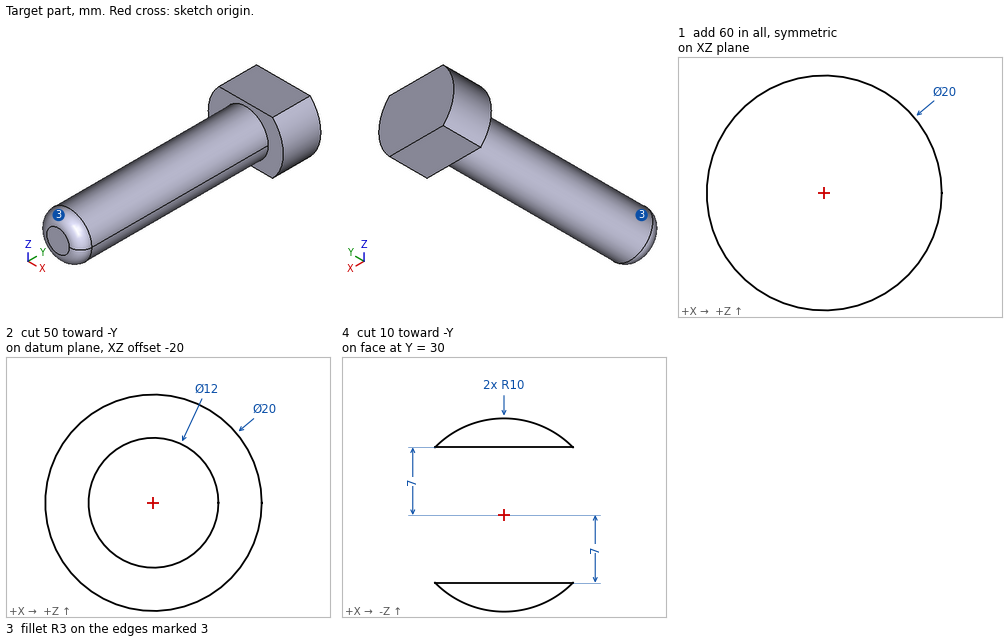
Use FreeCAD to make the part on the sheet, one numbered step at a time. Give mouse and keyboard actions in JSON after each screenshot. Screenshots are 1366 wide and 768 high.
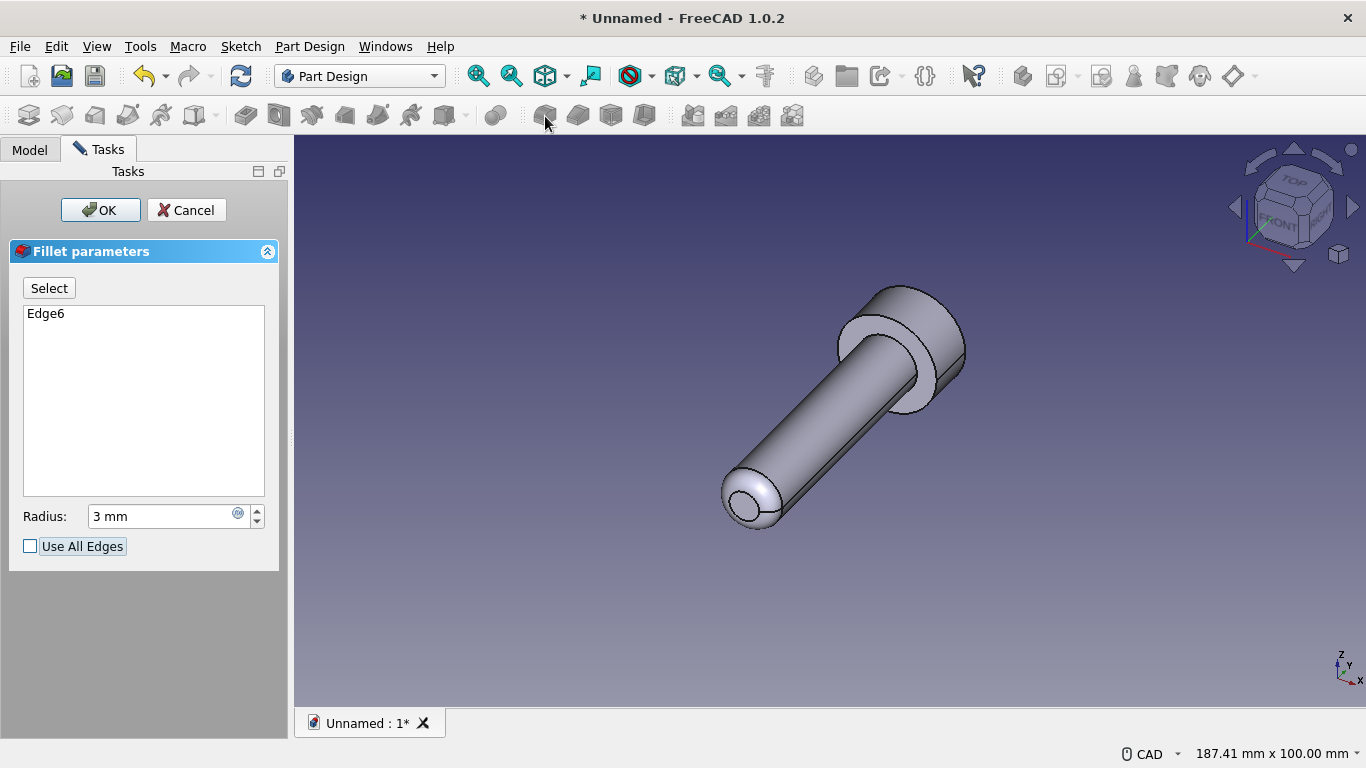
{"action": "left_click", "coordinate": [101, 210]}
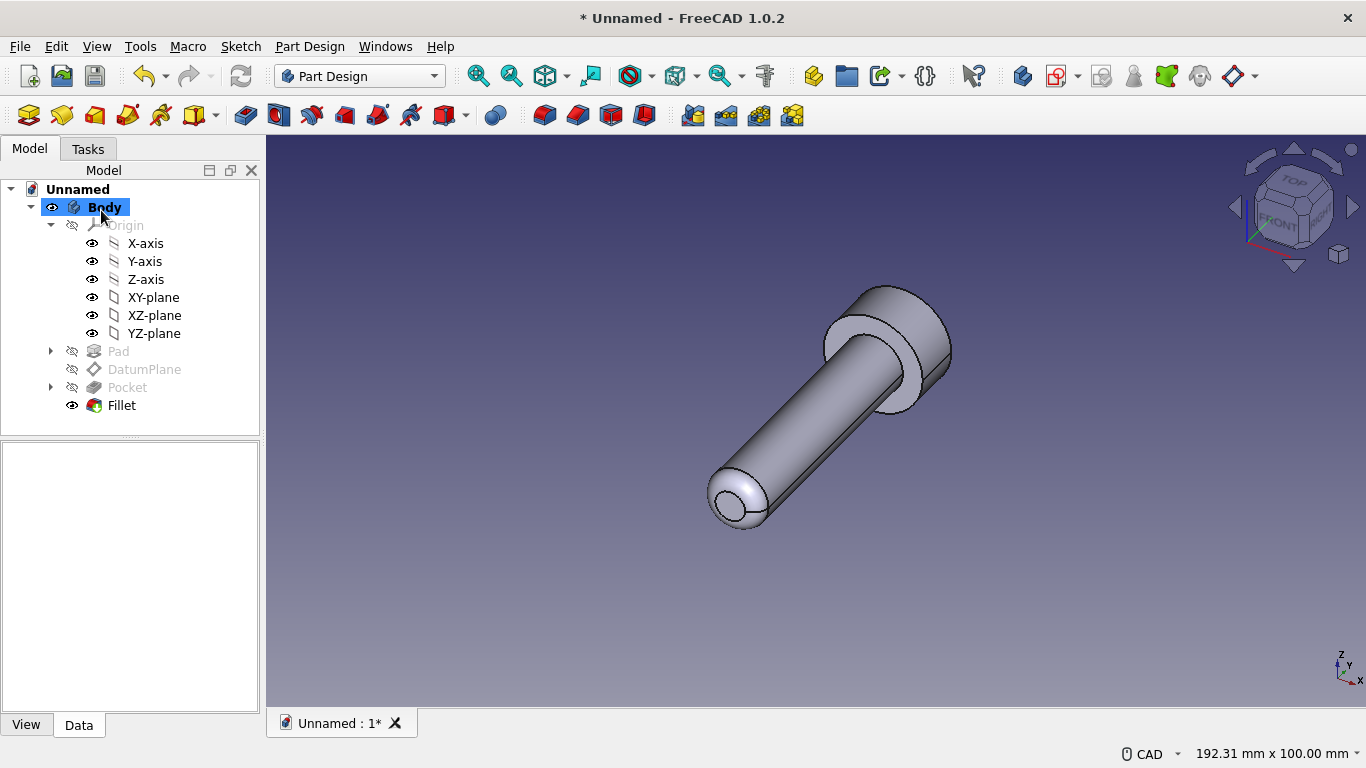
{"action": "key", "text": "4"}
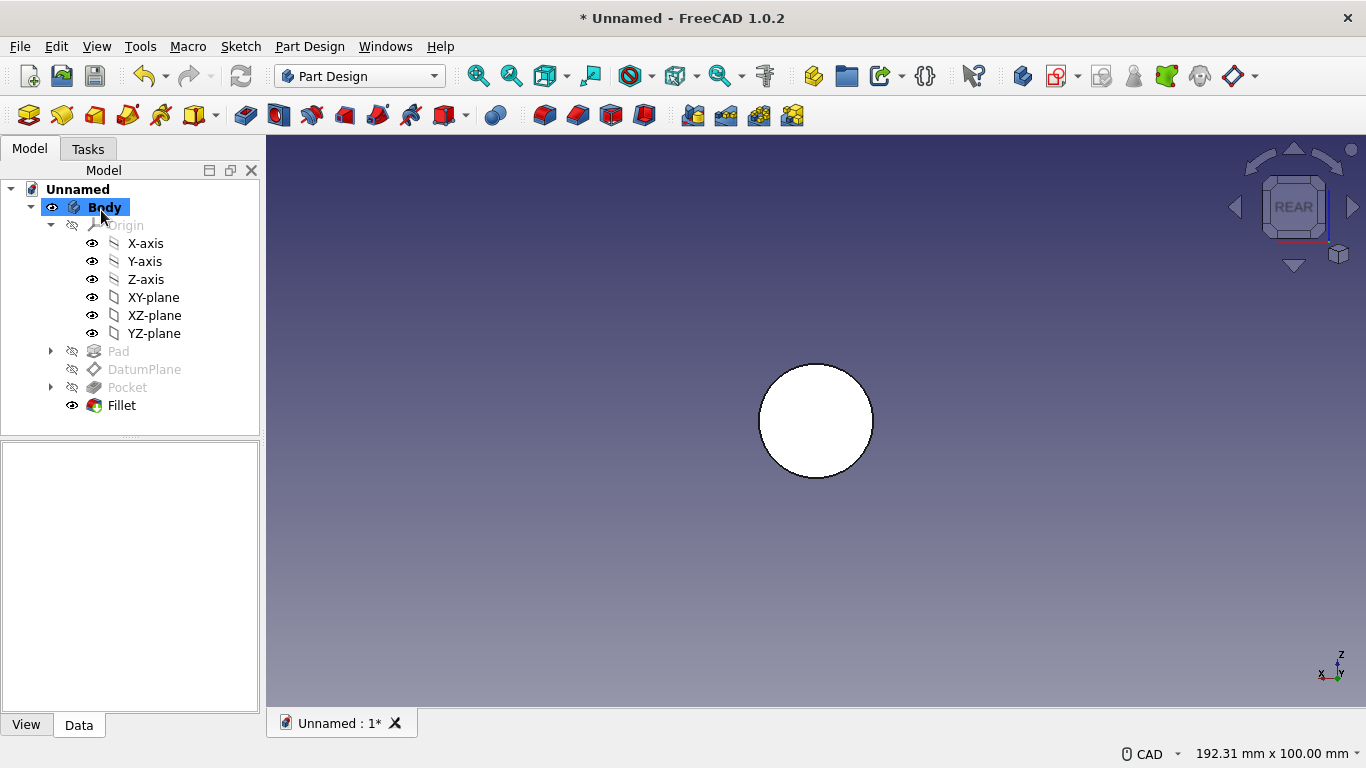
{"action": "left_click", "coordinate": [479, 76]}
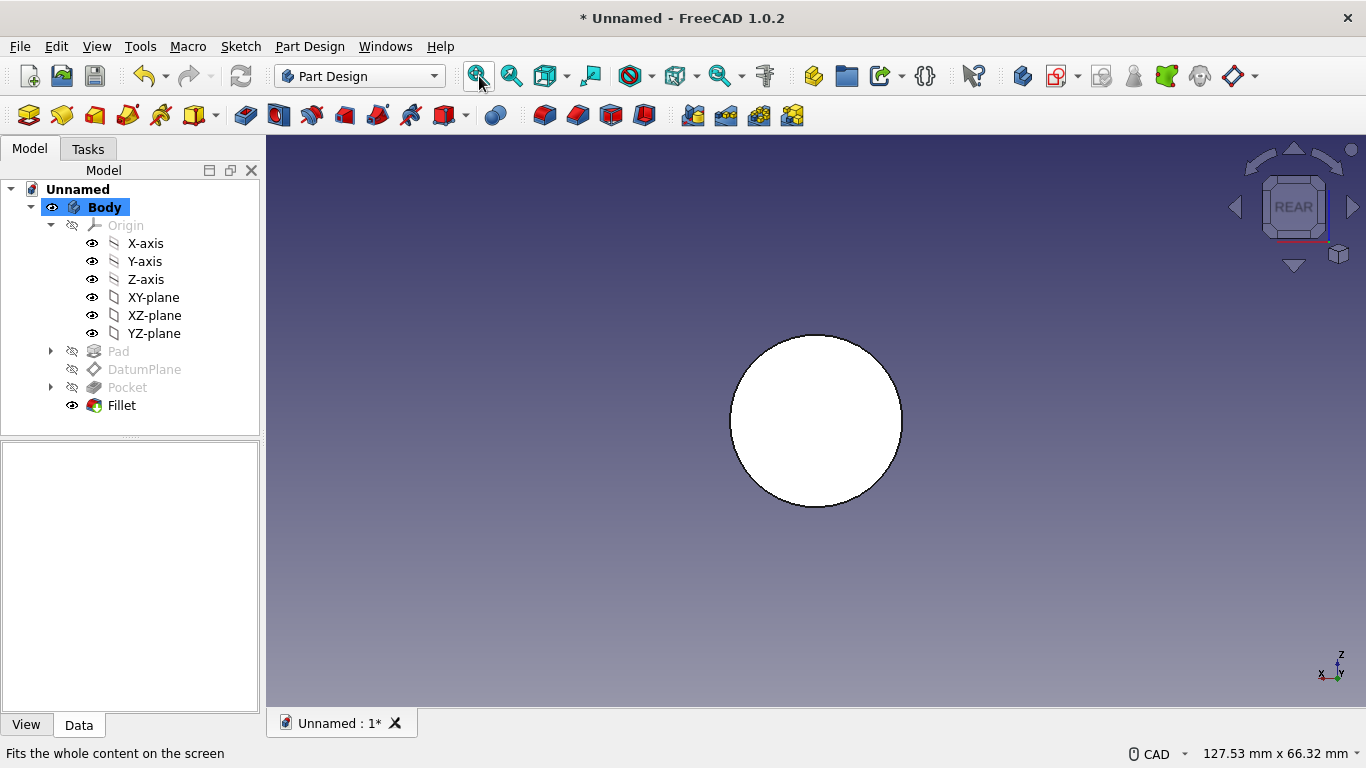
{"action": "left_click", "coordinate": [816, 420]}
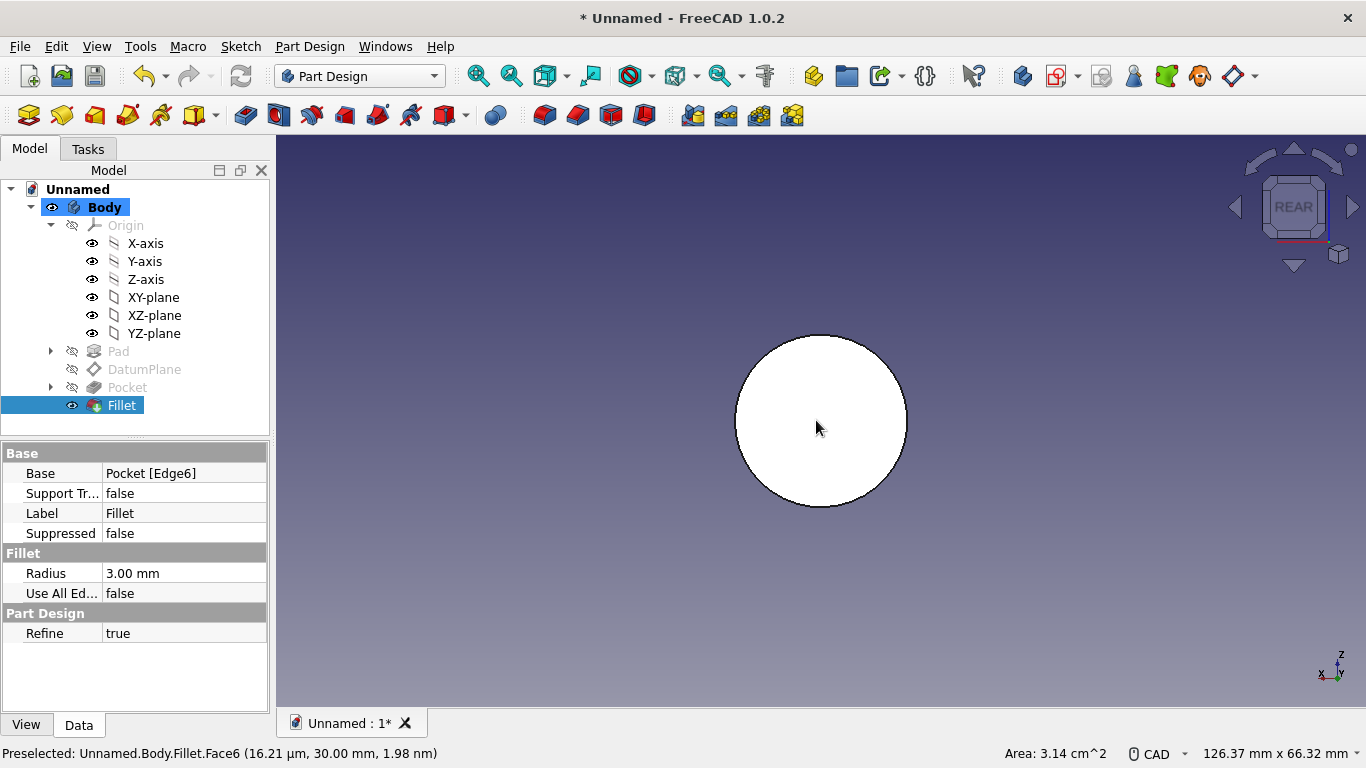
{"action": "left_click", "coordinate": [1056, 76]}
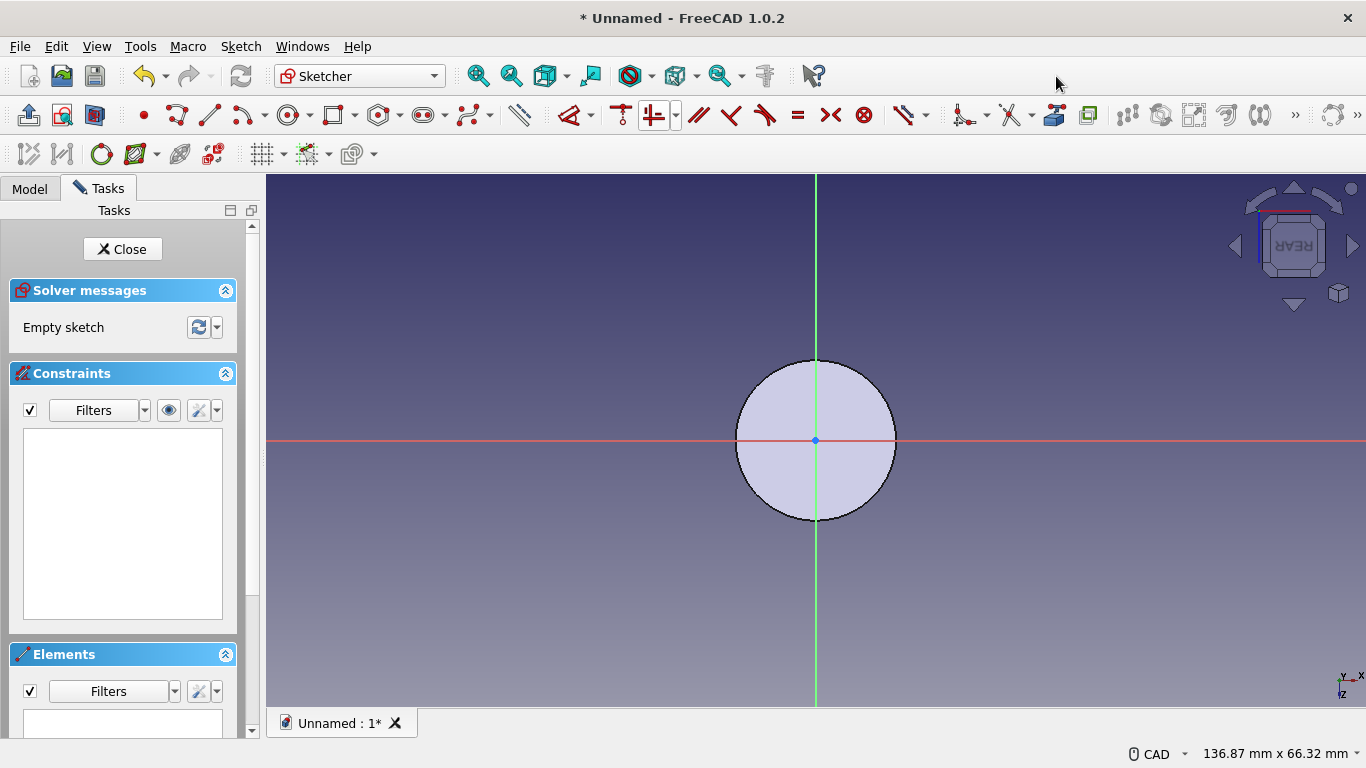
{"action": "scroll", "coordinate": [872, 440], "scroll_direction": "up", "scroll_amount": 4}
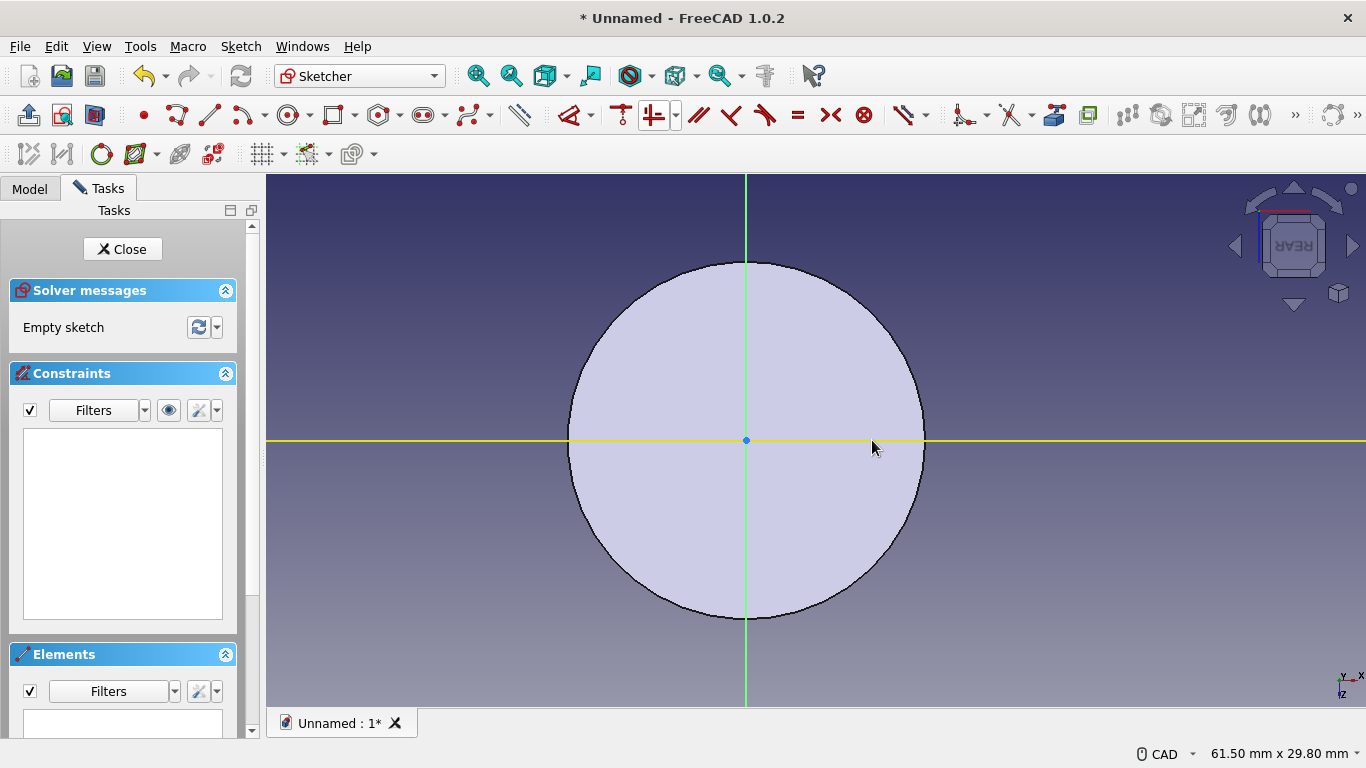
{"action": "left_click", "coordinate": [210, 116]}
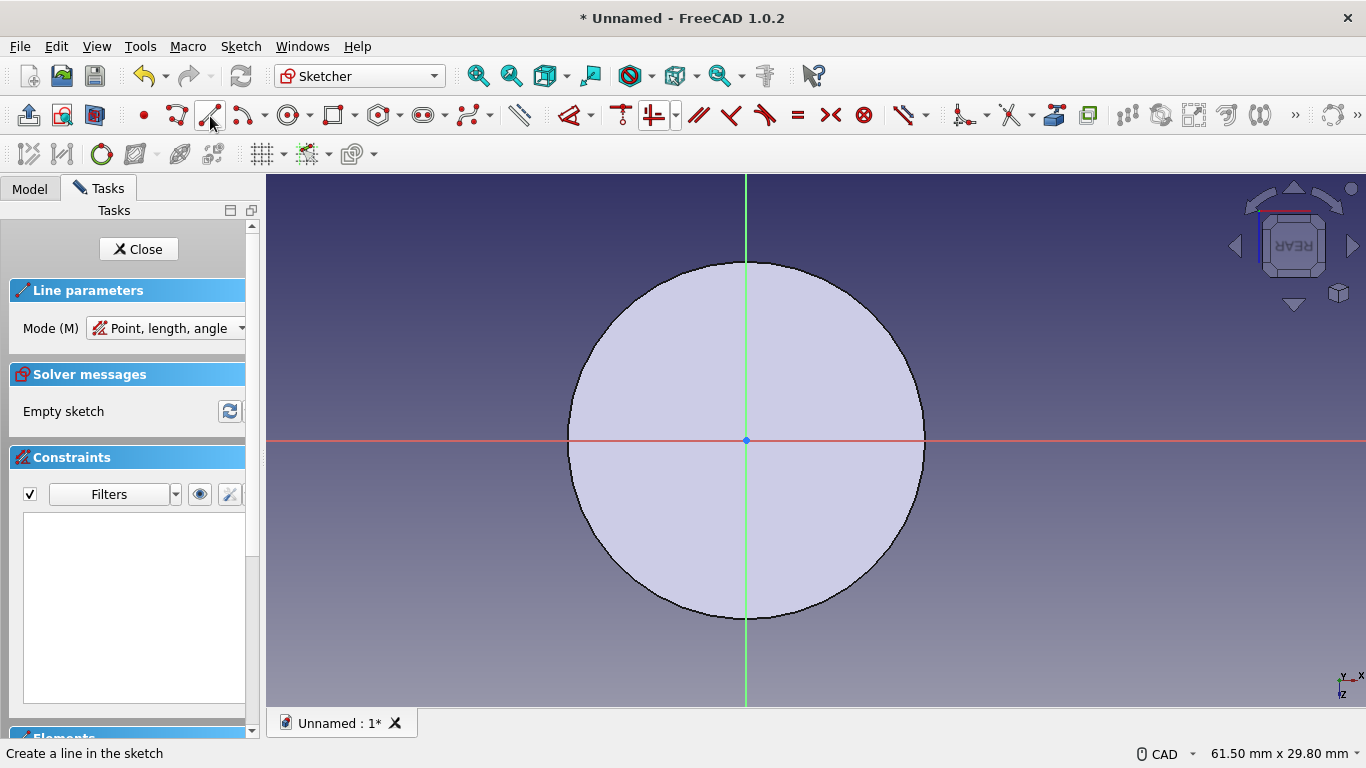
{"action": "left_click", "coordinate": [619, 315]}
{"action": "left_click", "coordinate": [874, 315]}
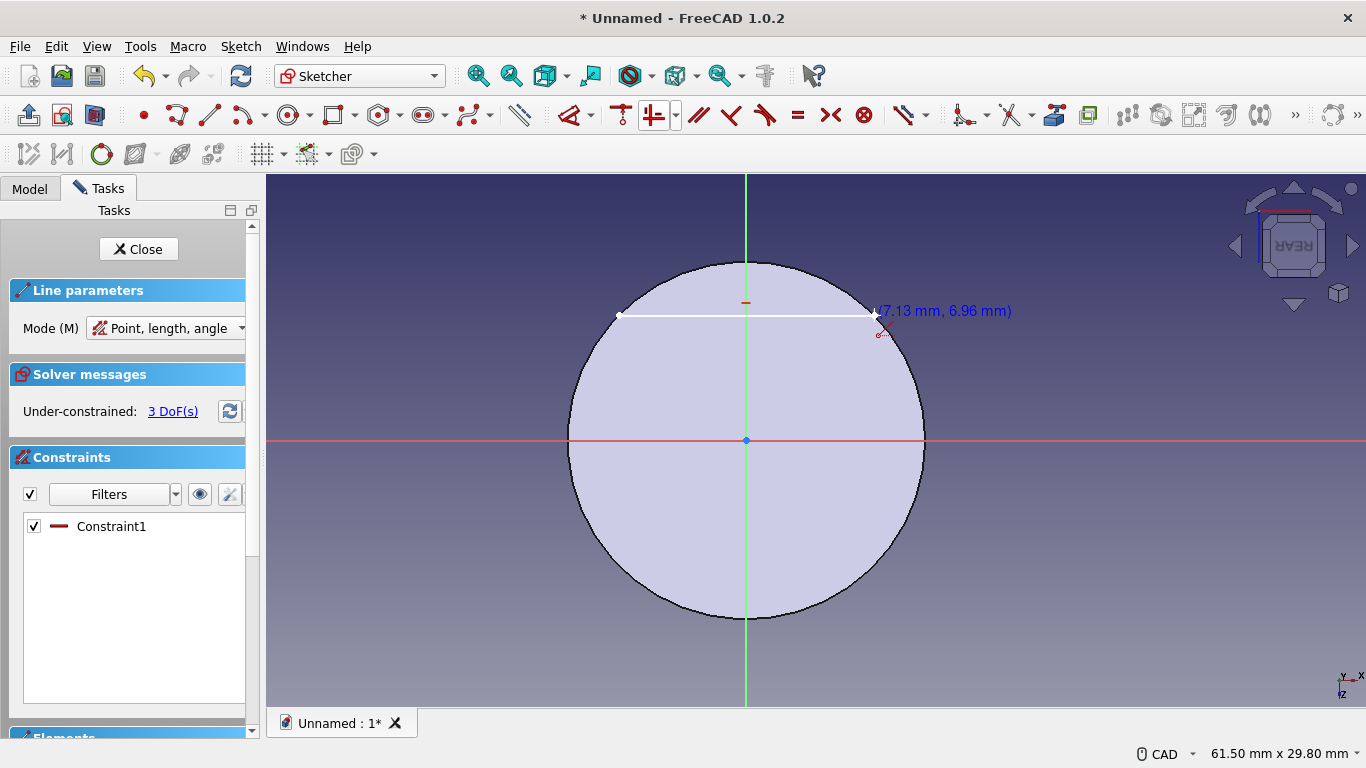
{"action": "key", "text": "g 3 a"}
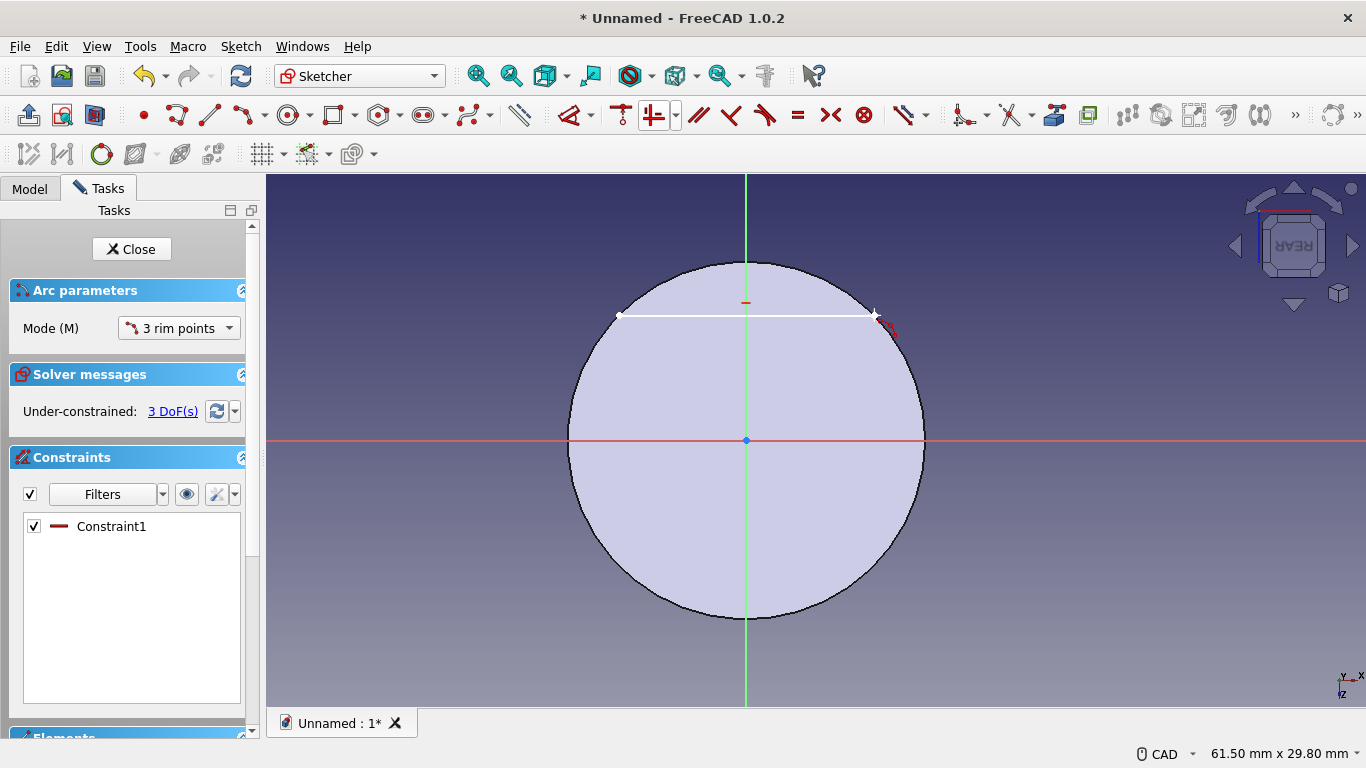
{"action": "left_click", "coordinate": [874, 316]}
{"action": "left_click", "coordinate": [619, 316]}
{"action": "left_click", "coordinate": [775, 264]}